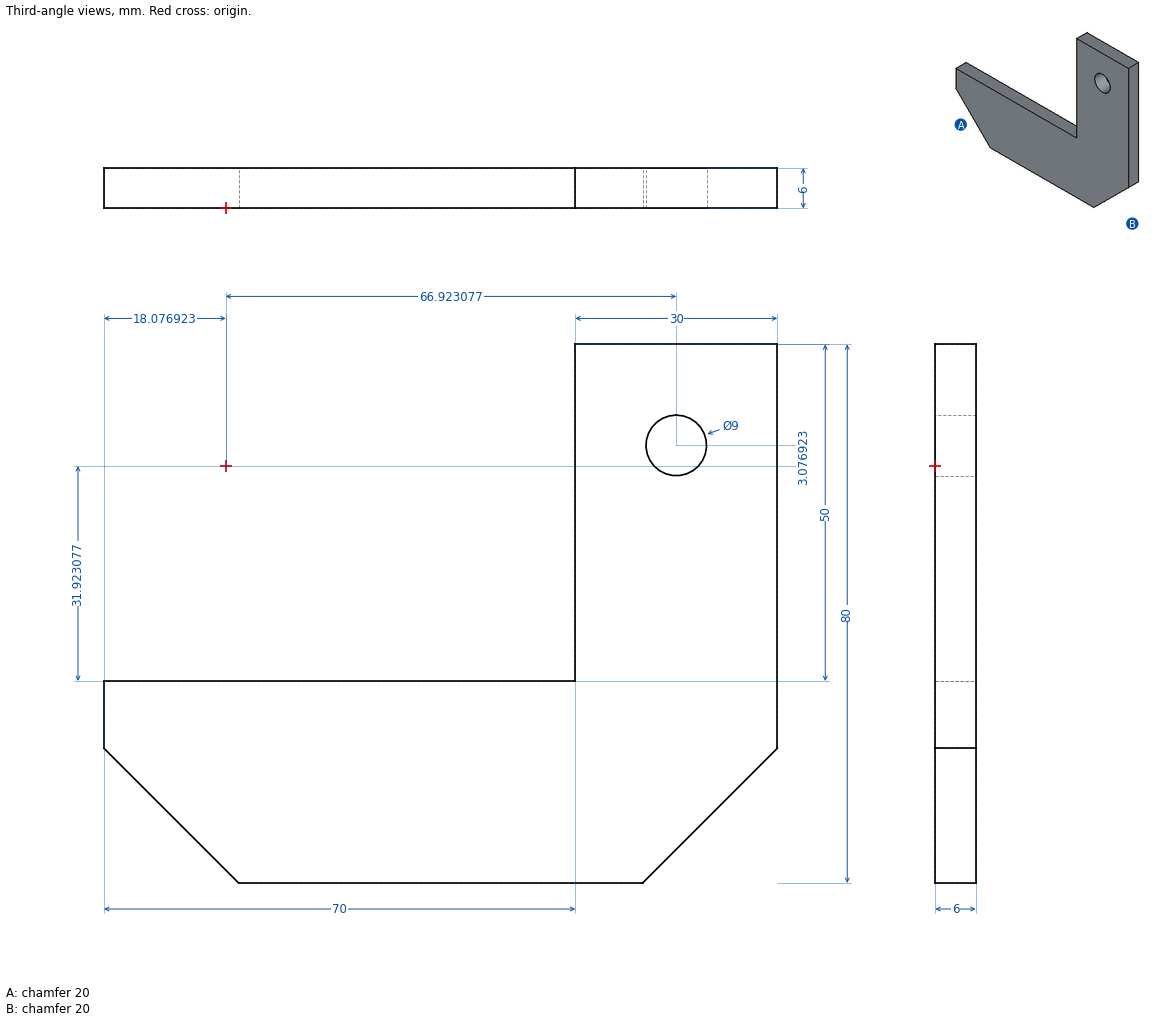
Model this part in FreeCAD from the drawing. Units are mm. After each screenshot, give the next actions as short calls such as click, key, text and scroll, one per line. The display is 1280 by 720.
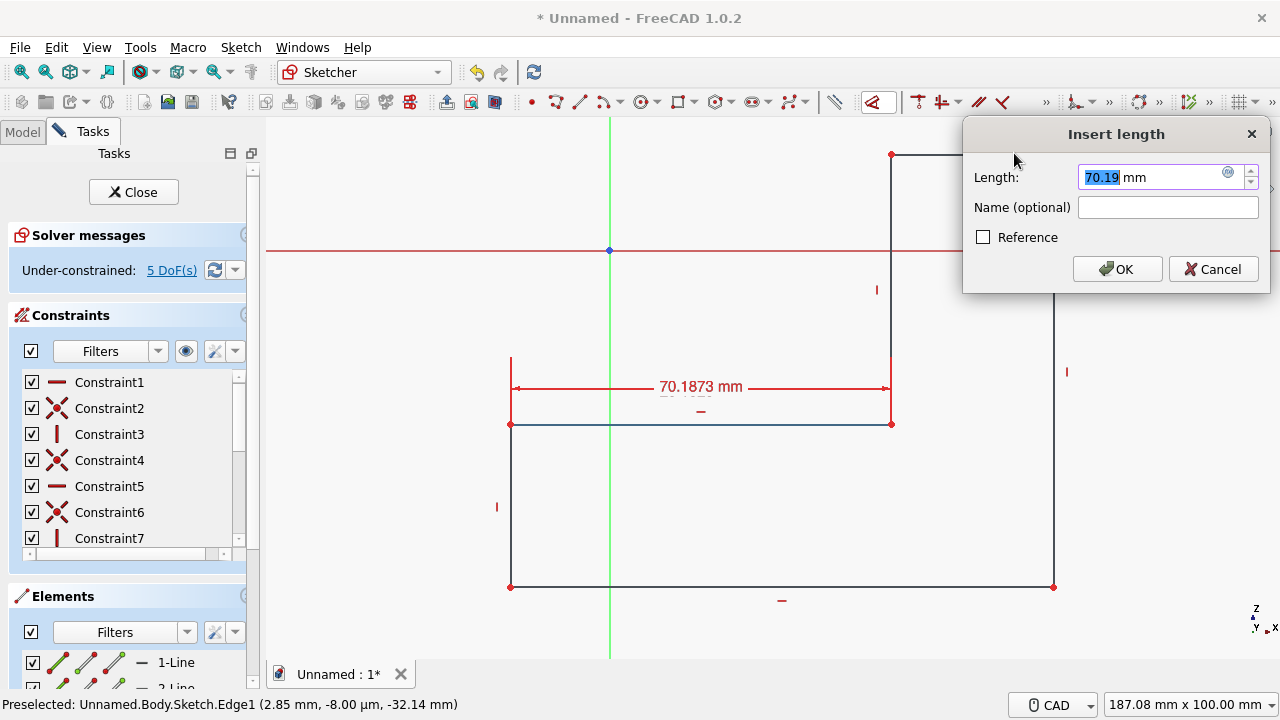
text(70)
key(Return)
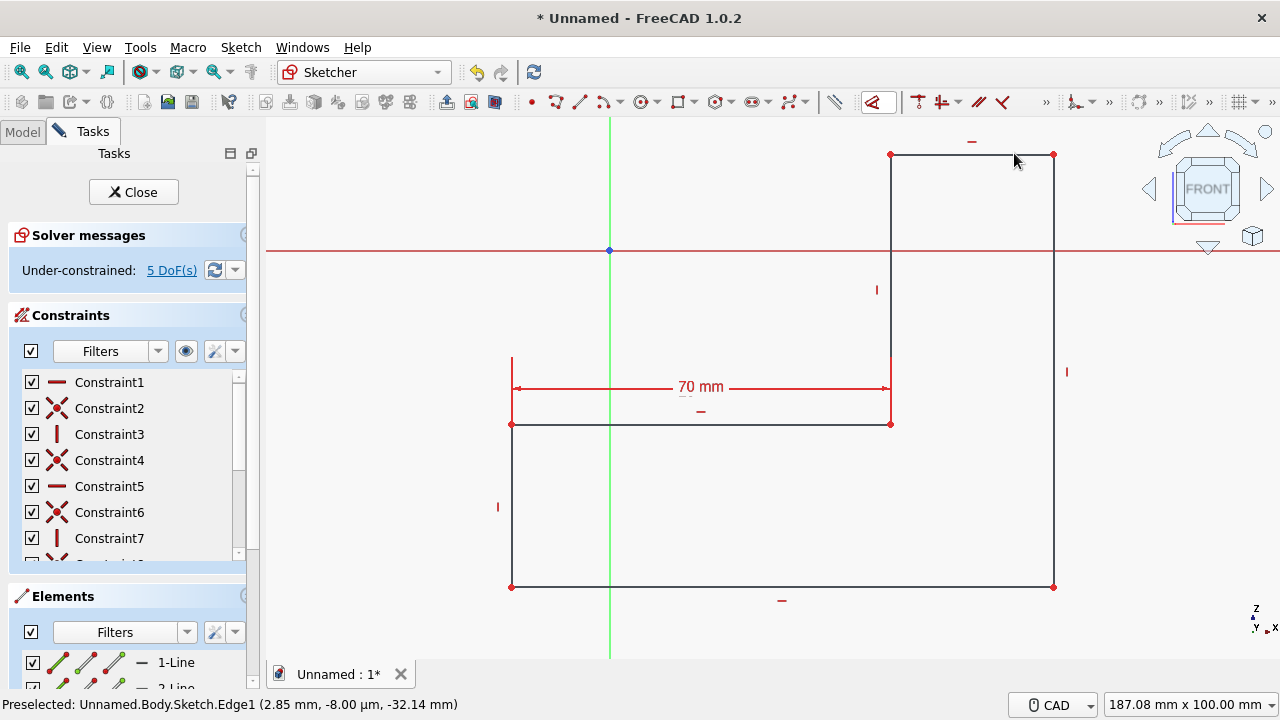
click(891, 344)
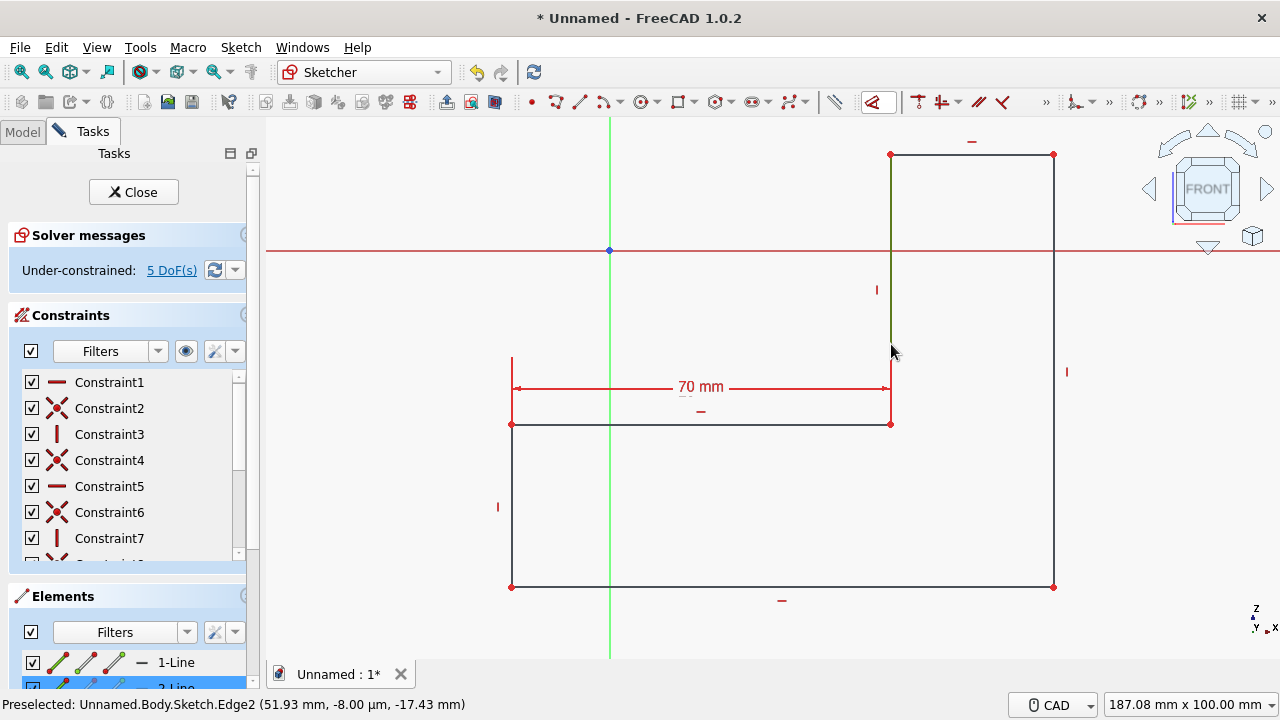
click(890, 102)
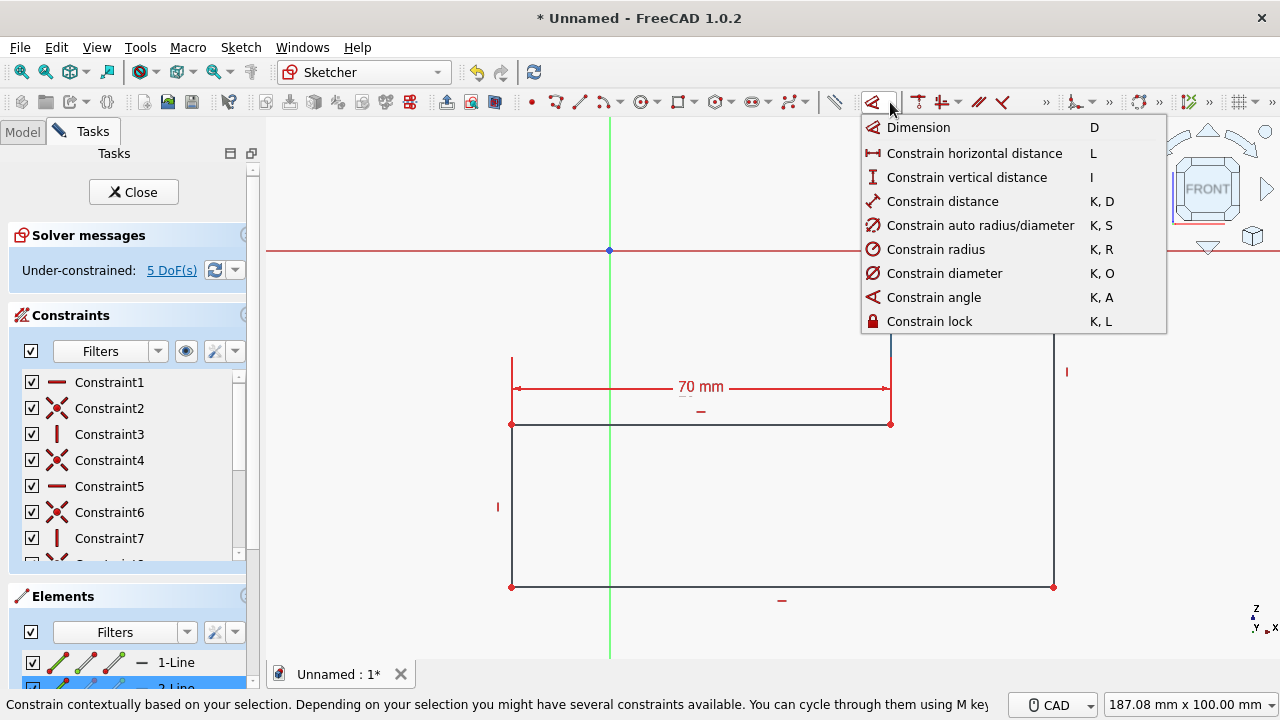
click(1014, 177)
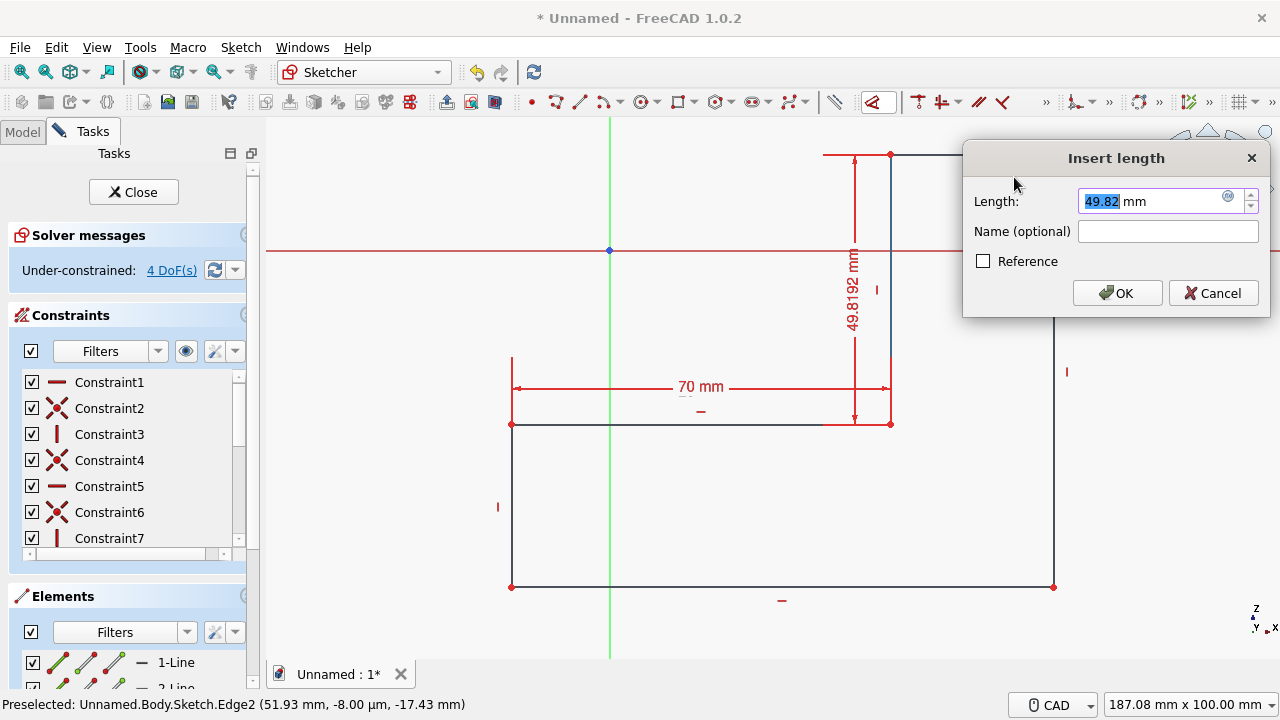
text(50)
key(Return)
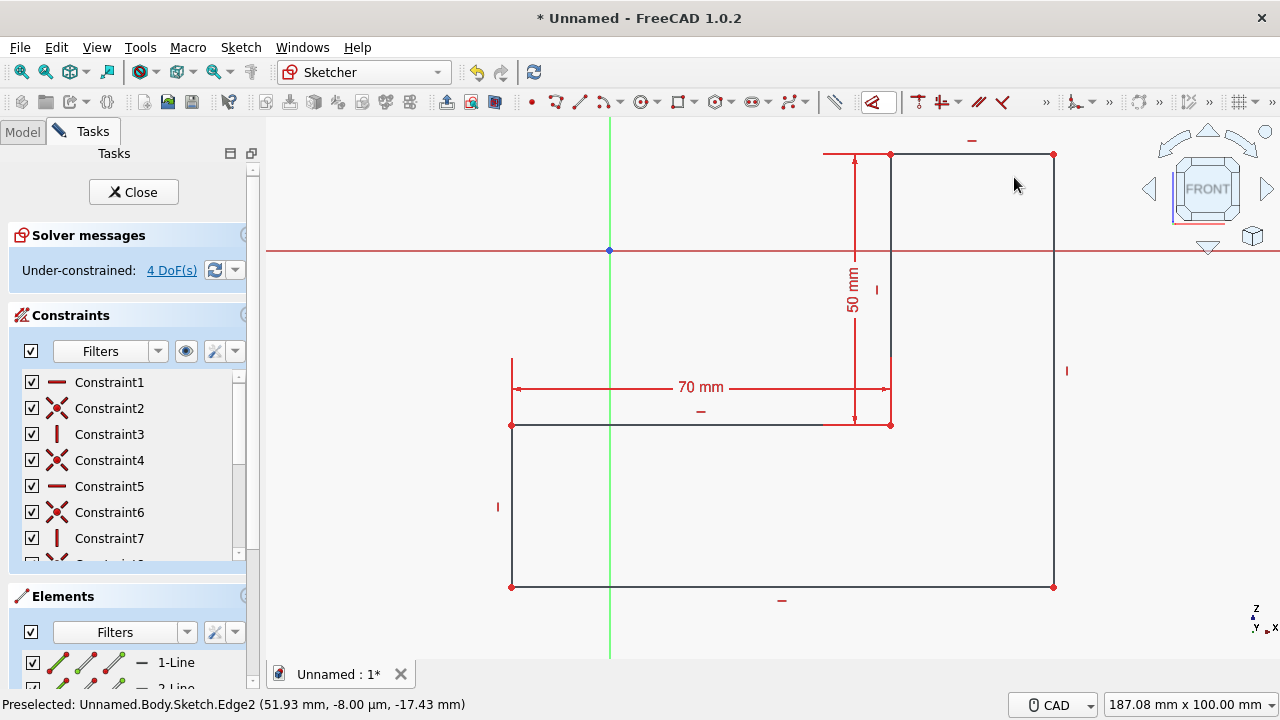
click(940, 154)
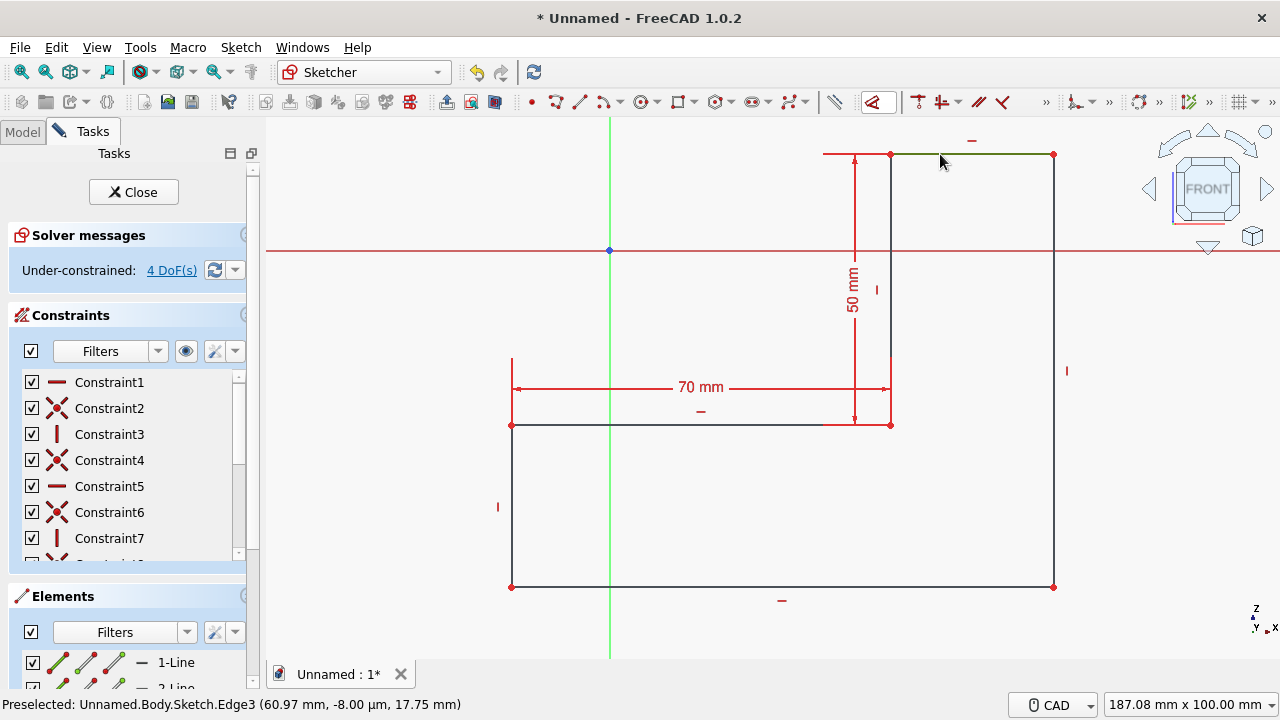
key(l)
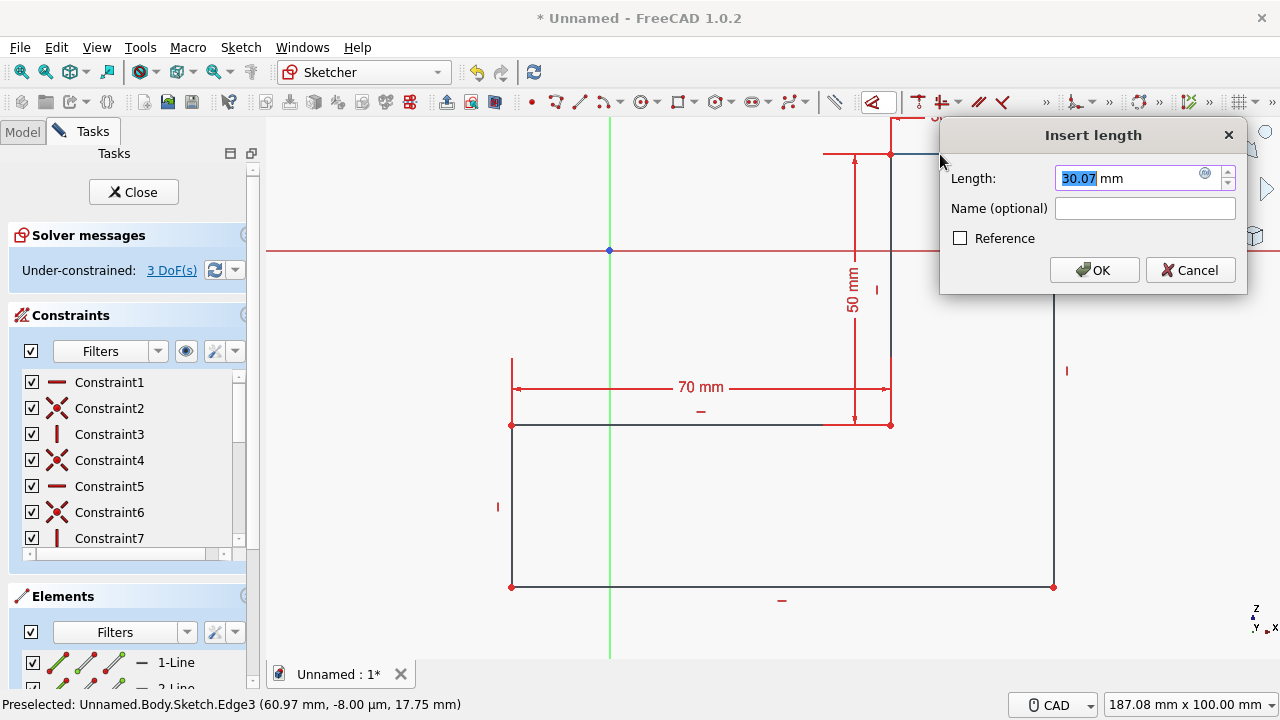
text(30)
key(Return)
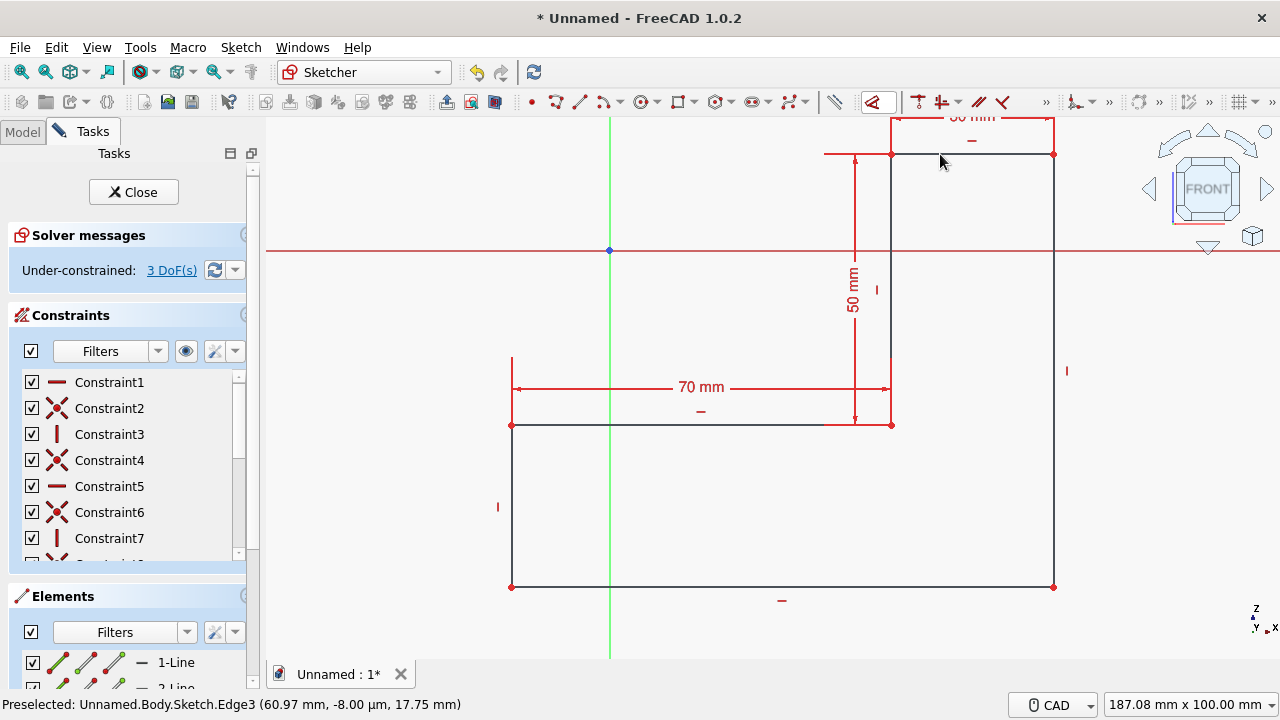
click(1054, 284)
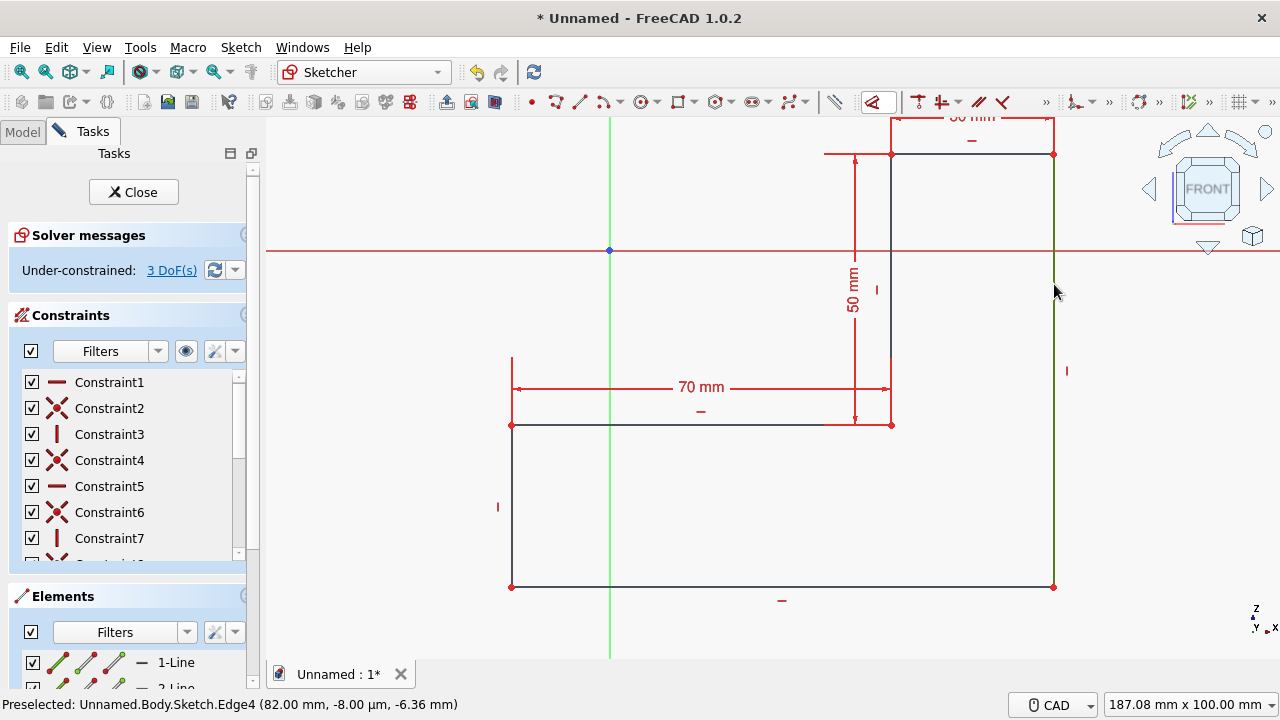
key(i)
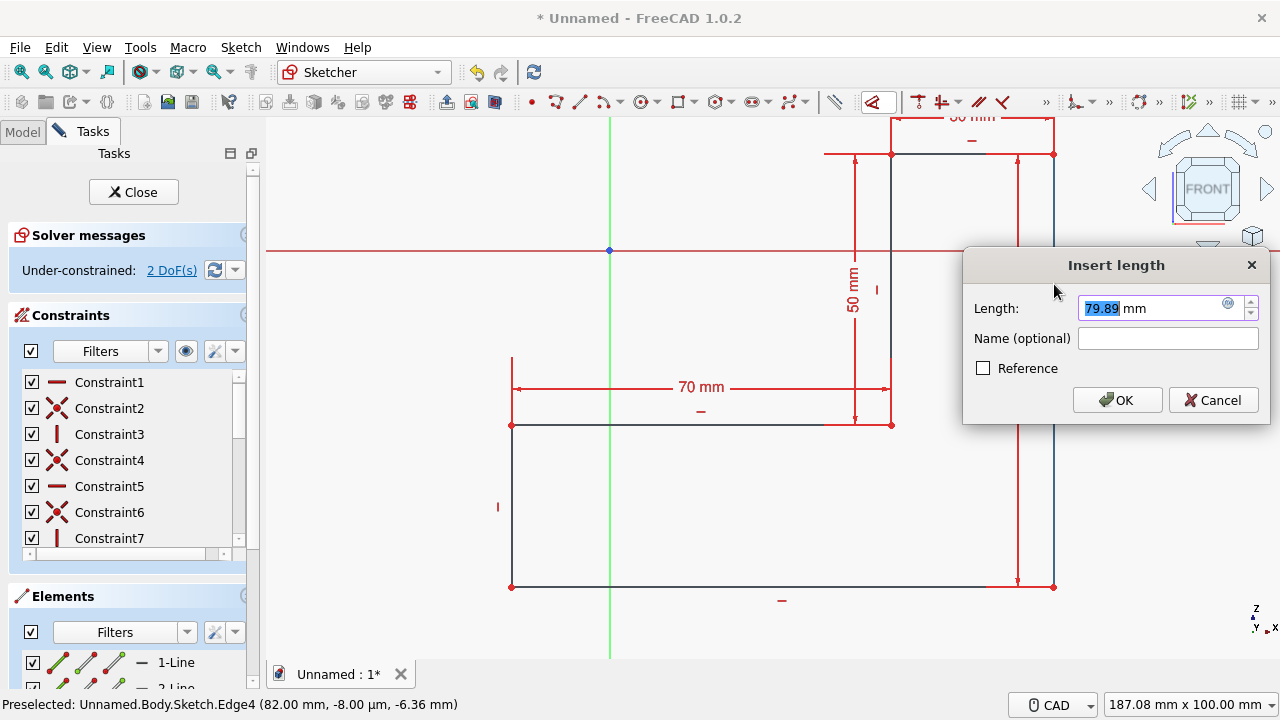
text(80)
key(Return)